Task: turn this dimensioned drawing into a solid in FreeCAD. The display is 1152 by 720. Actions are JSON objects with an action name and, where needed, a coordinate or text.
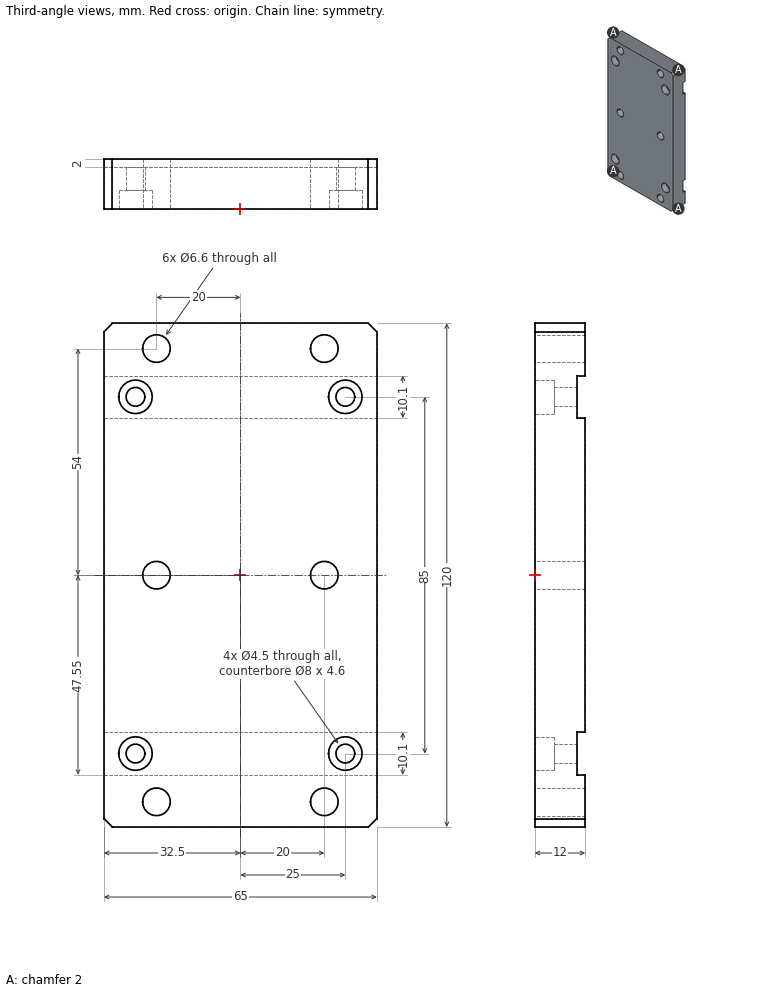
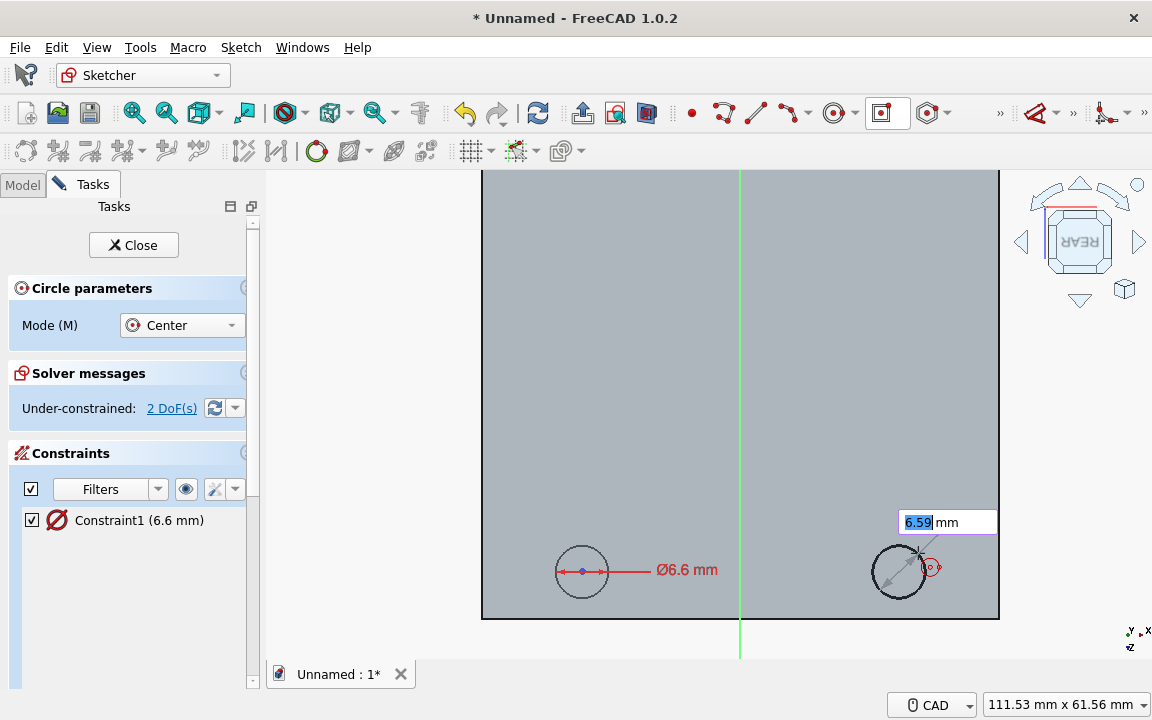
{"action": "type", "text": "6.6"}
{"action": "key", "text": "Return"}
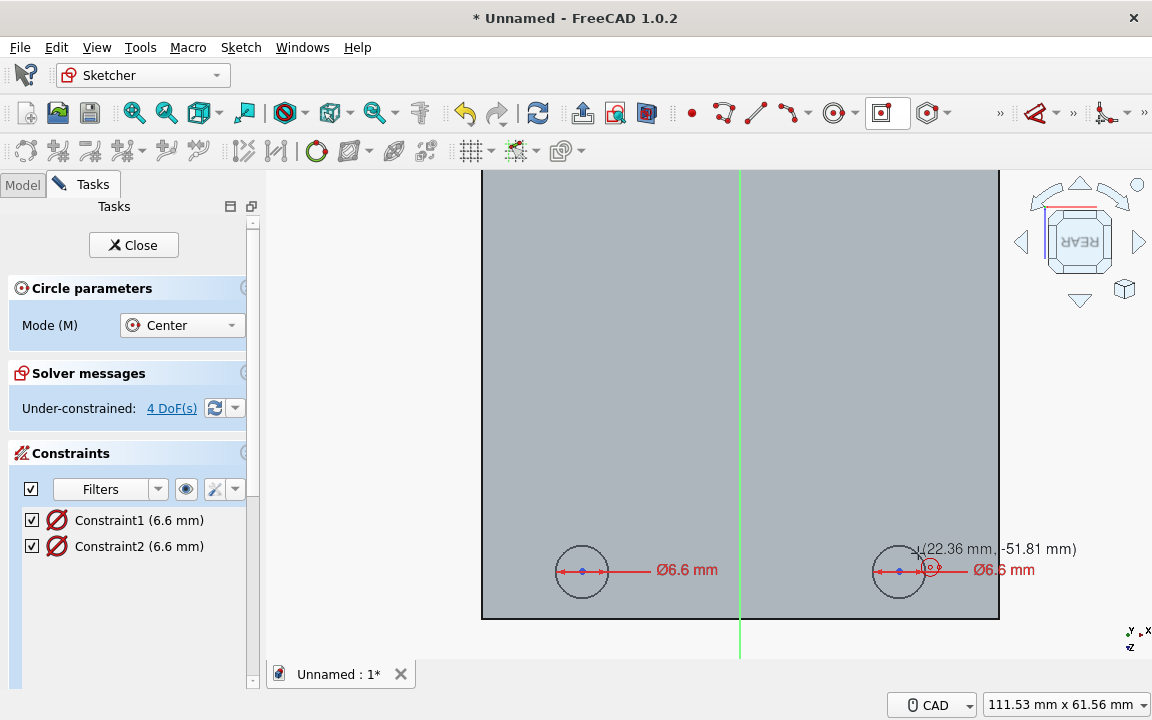
{"action": "scroll", "coordinate": [582, 573], "scroll_direction": "down", "scroll_amount": 5}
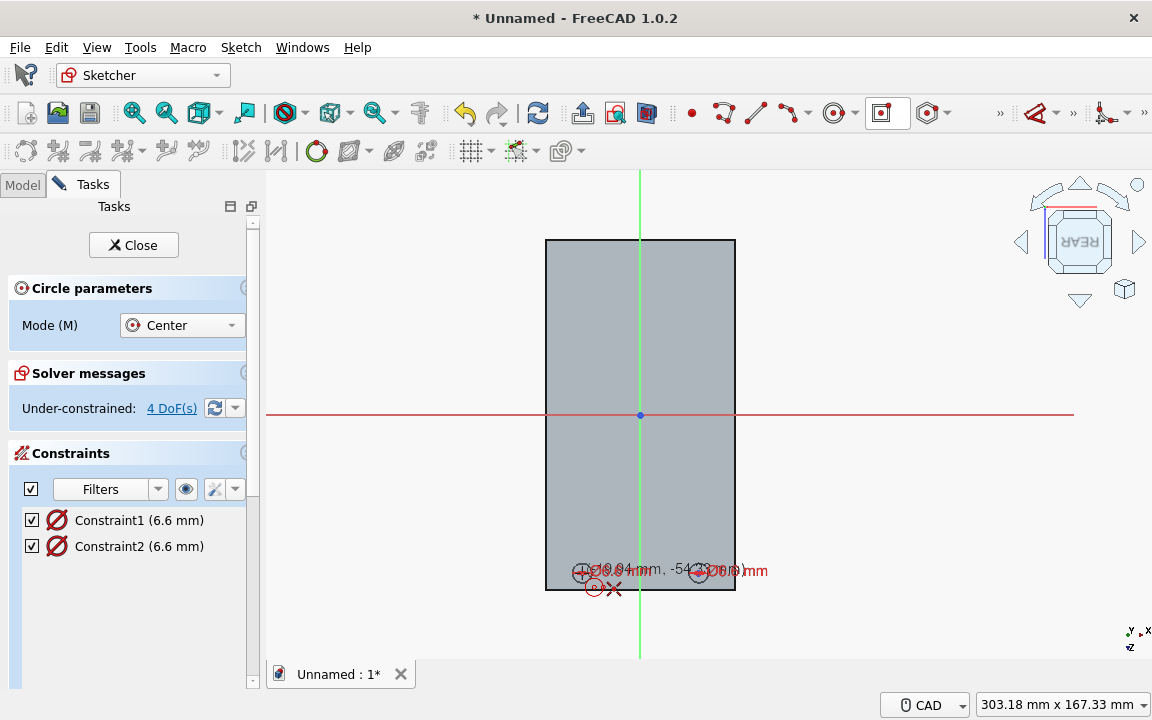
{"action": "scroll", "coordinate": [582, 415], "scroll_direction": "up", "scroll_amount": 5}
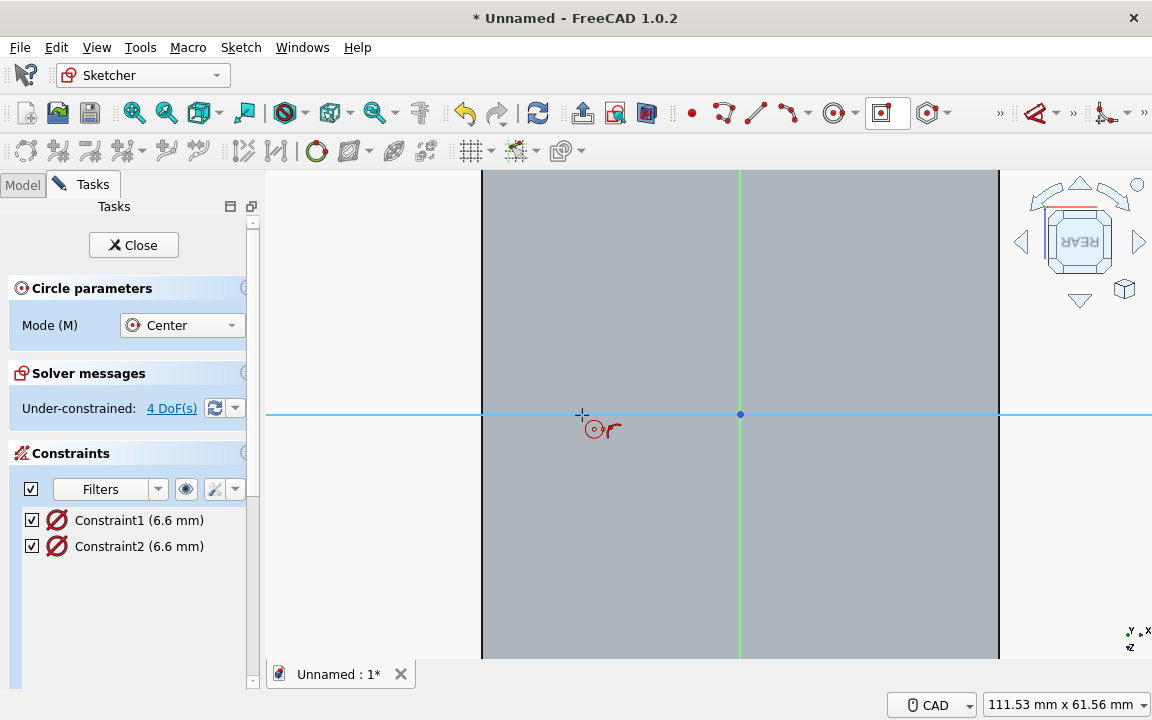
{"action": "left_click", "coordinate": [582, 415]}
{"action": "mouse_move", "coordinate": [600, 396]}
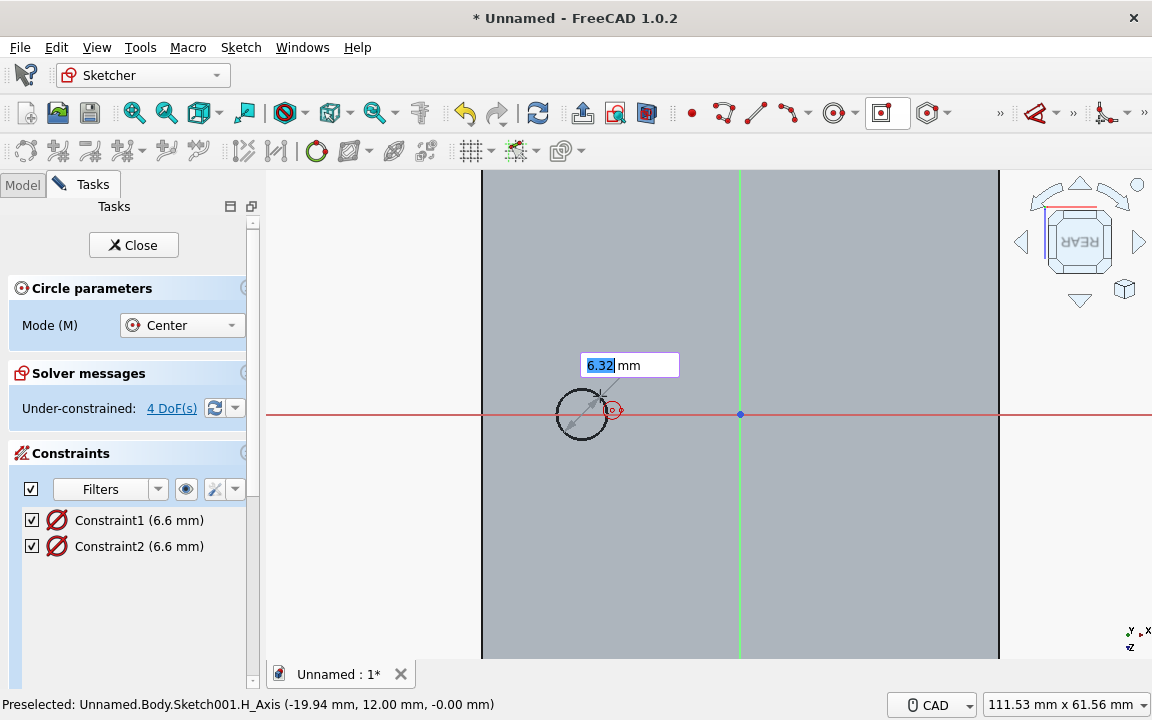
{"action": "type", "text": "6.6"}
{"action": "key", "text": "Return"}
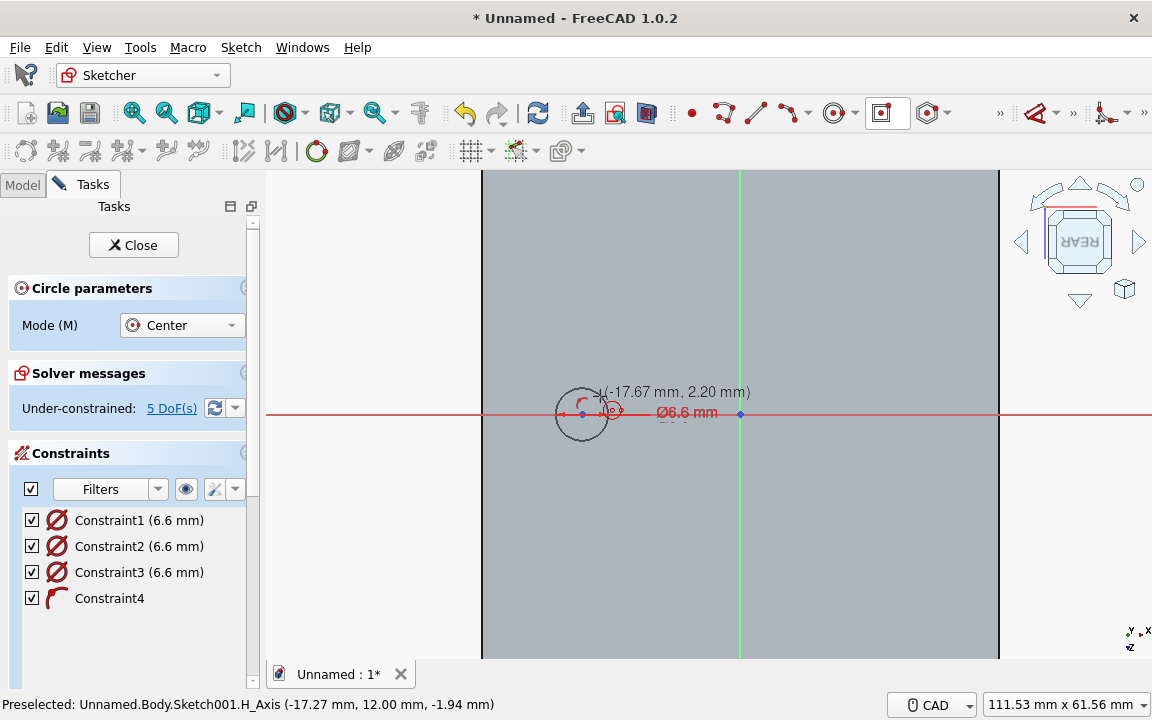
{"action": "left_click", "coordinate": [899, 415]}
{"action": "mouse_move", "coordinate": [918, 396]}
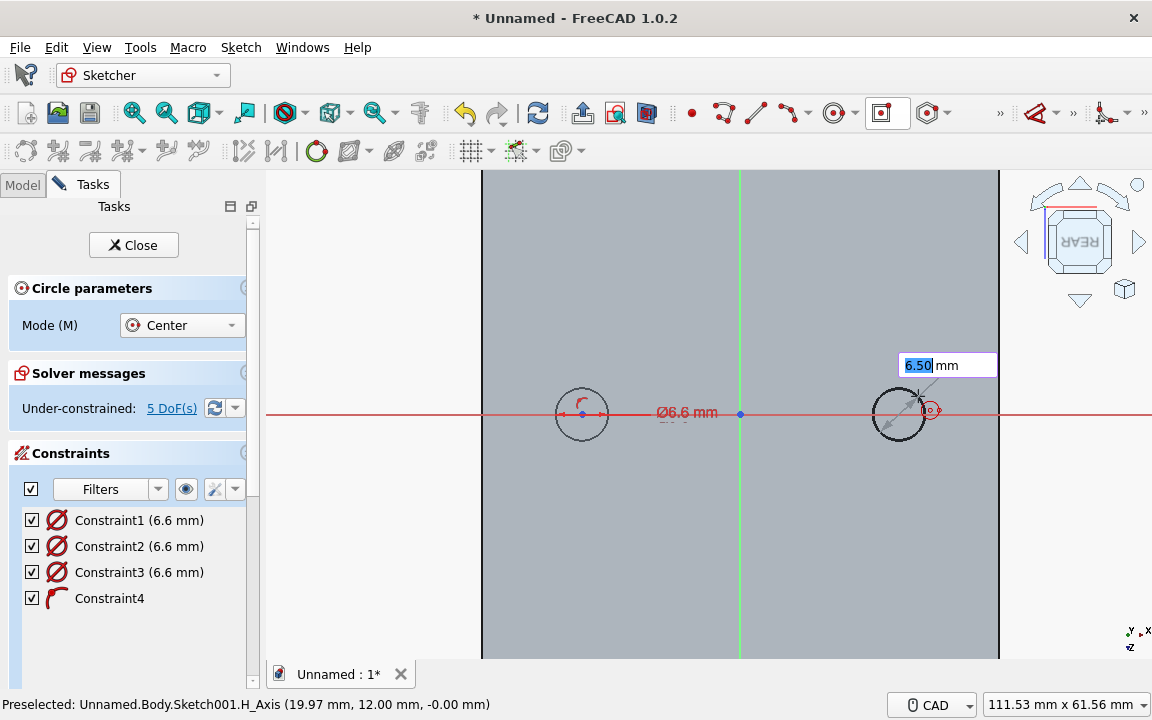
{"action": "type", "text": "6.6"}
{"action": "key", "text": "Return"}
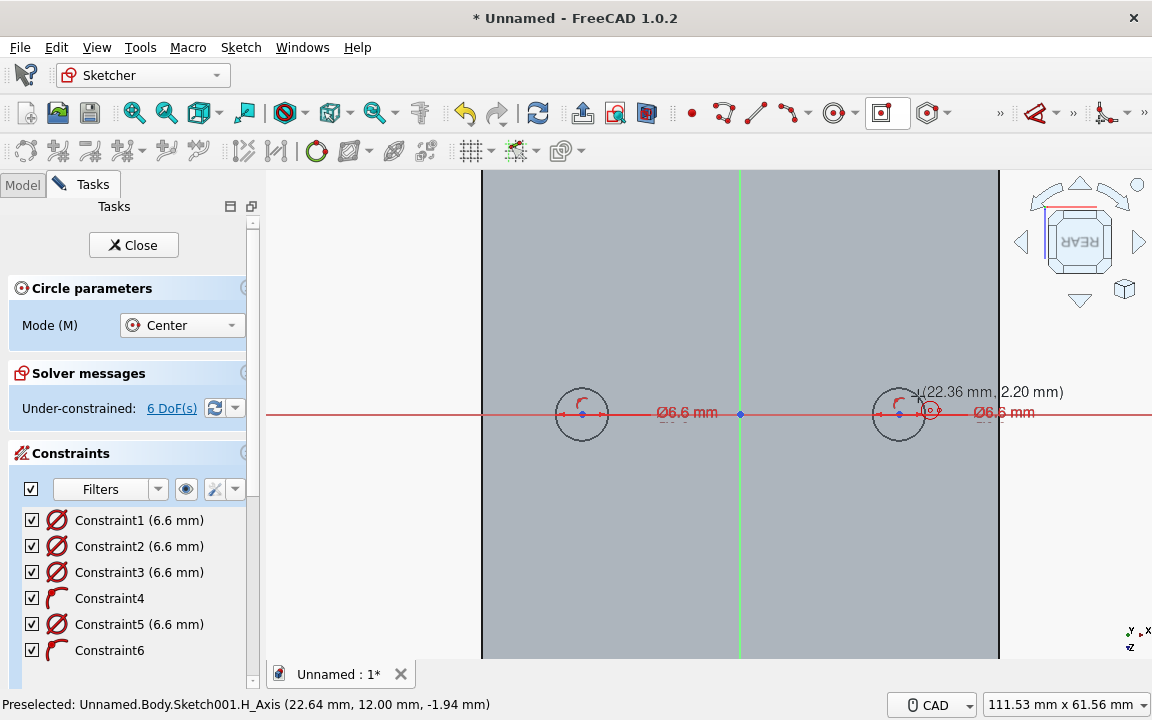
{"action": "scroll", "coordinate": [582, 414], "scroll_direction": "down", "scroll_amount": 5}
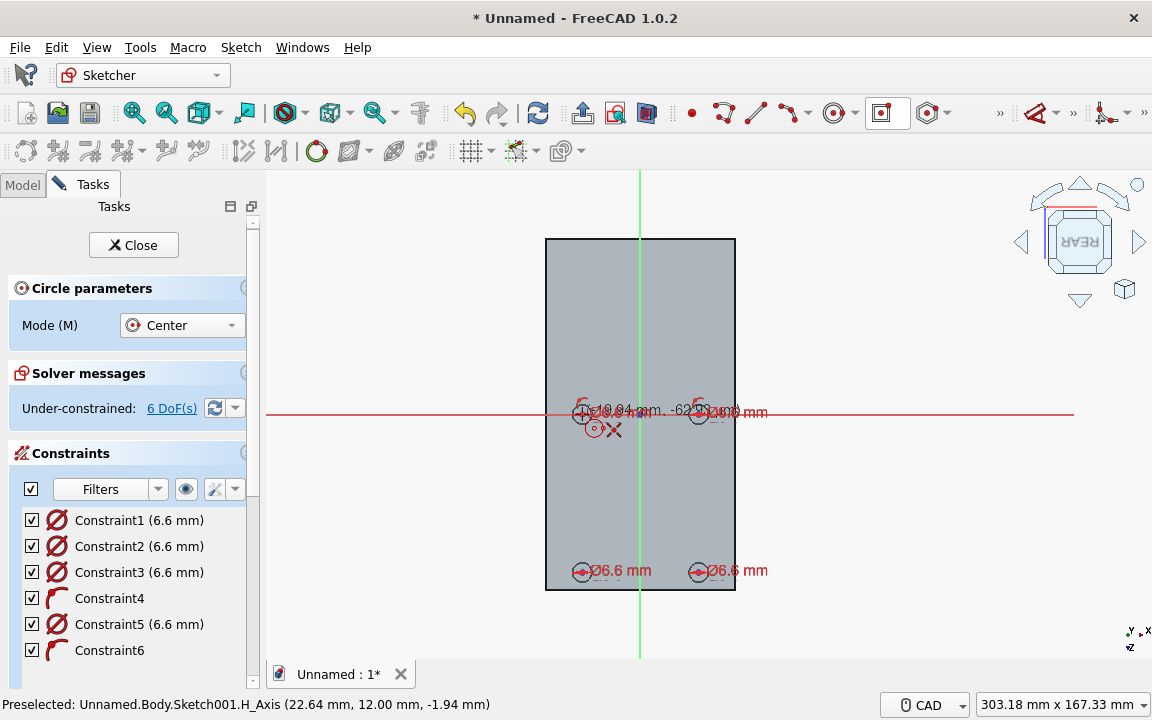
{"action": "scroll", "coordinate": [582, 257], "scroll_direction": "up", "scroll_amount": 5}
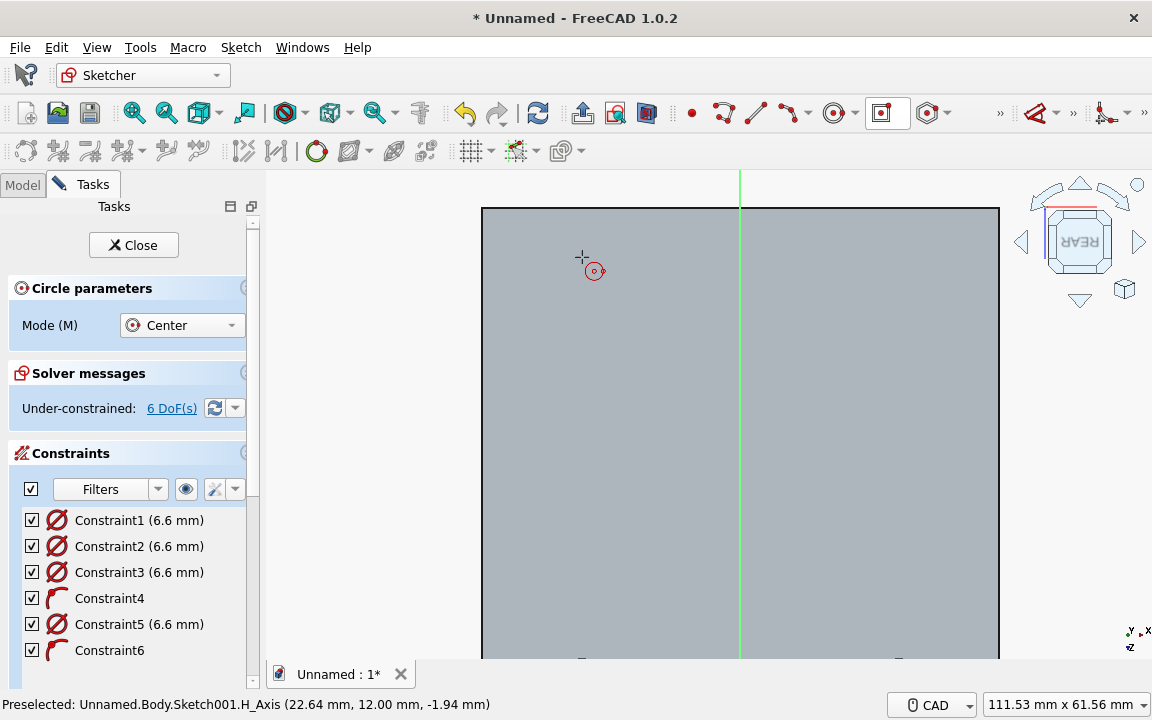
{"action": "left_click", "coordinate": [582, 256]}
{"action": "mouse_move", "coordinate": [600, 237]}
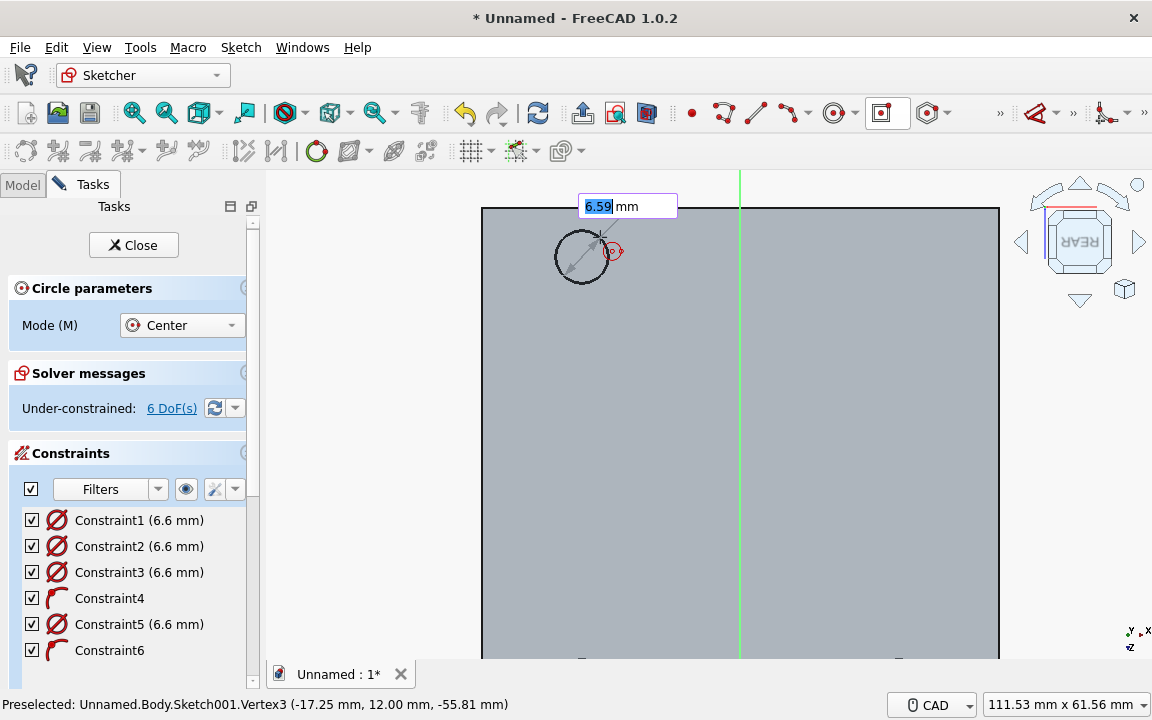
{"action": "type", "text": "6.6"}
{"action": "key", "text": "Return"}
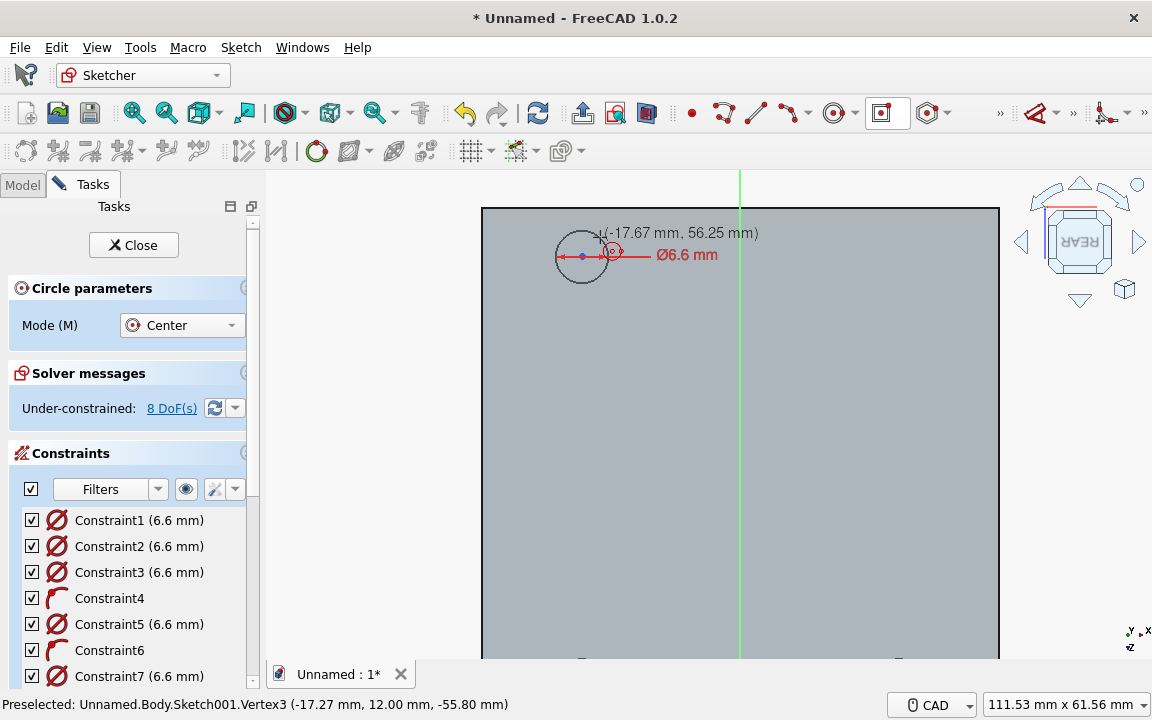
{"action": "left_click", "coordinate": [899, 256]}
{"action": "mouse_move", "coordinate": [918, 237]}